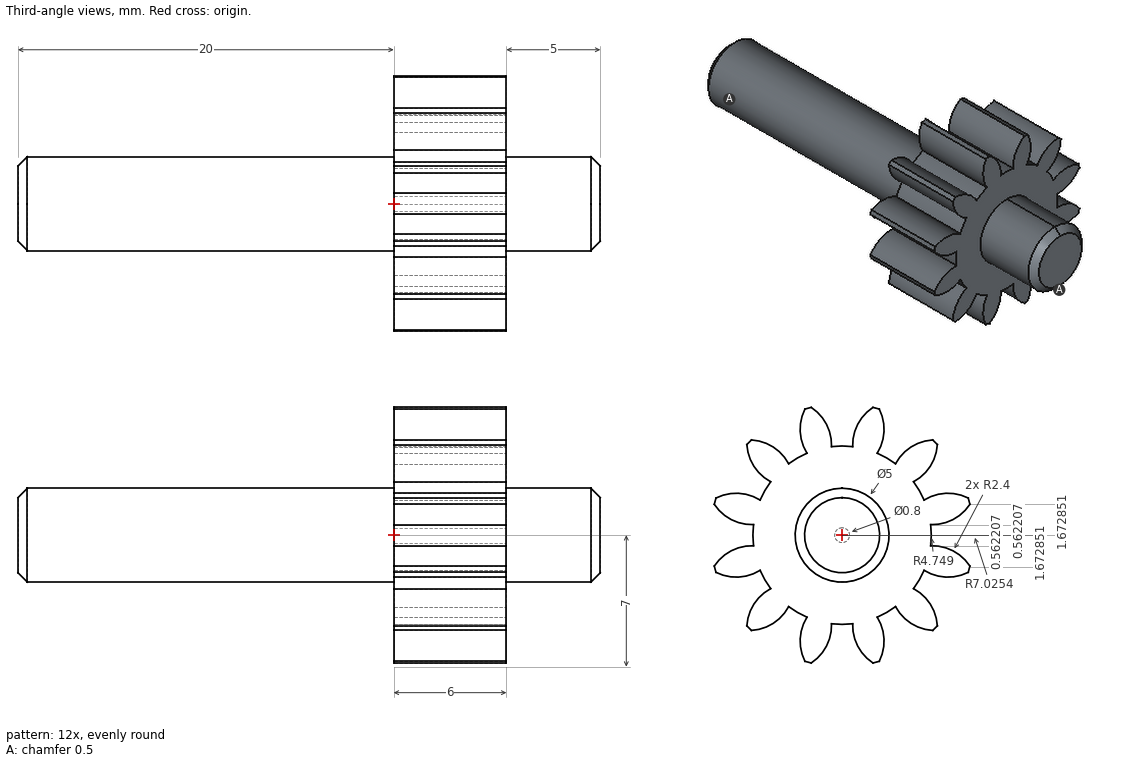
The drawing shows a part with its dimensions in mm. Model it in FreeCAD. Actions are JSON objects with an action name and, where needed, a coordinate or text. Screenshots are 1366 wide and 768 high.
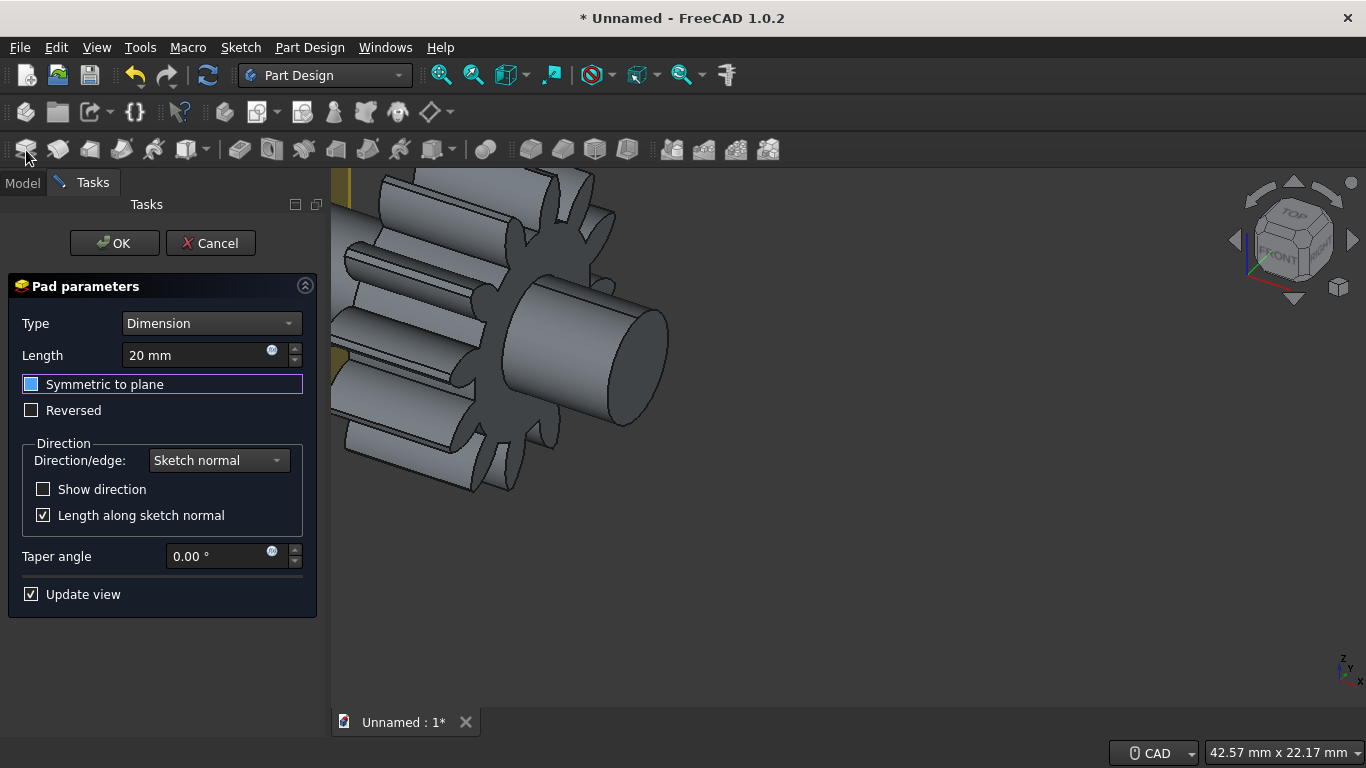
{"action": "left_click", "coordinate": [115, 243]}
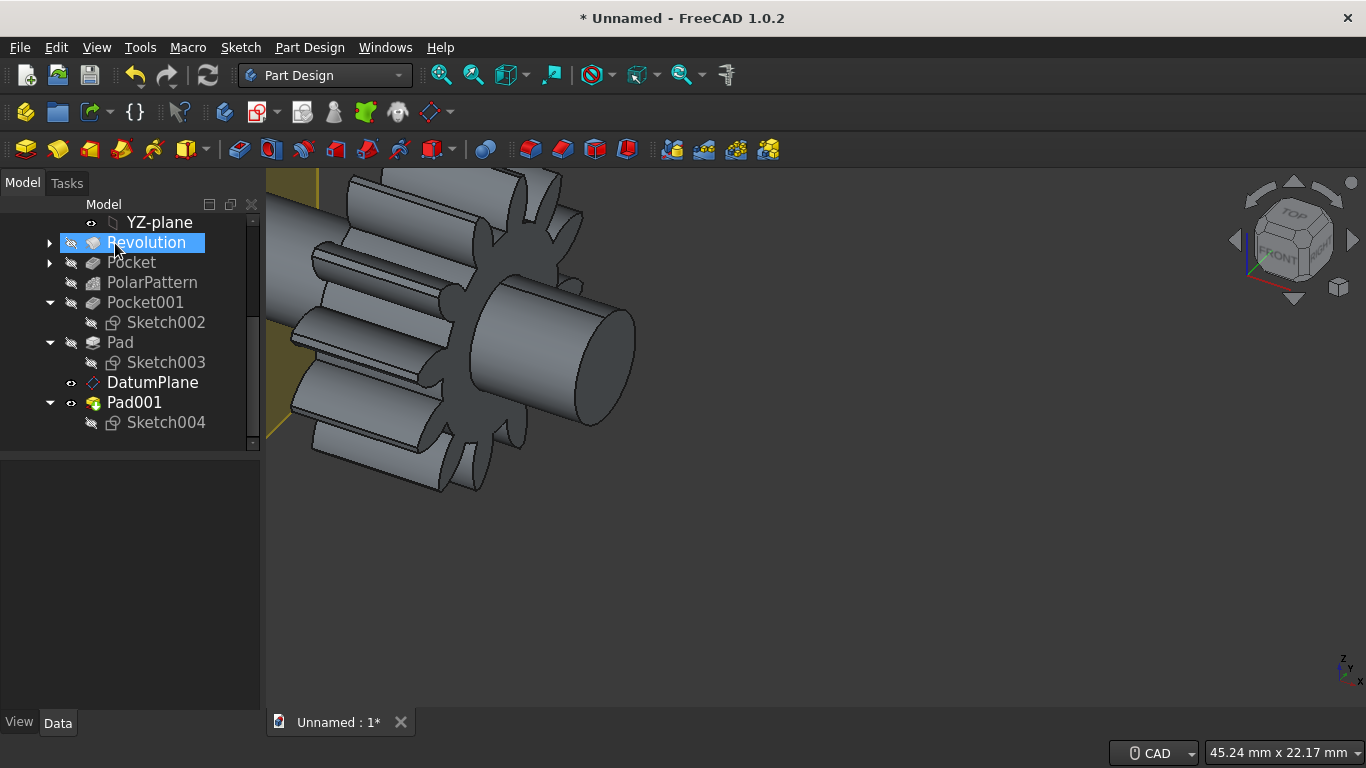
{"action": "left_click", "coordinate": [116, 383]}
{"action": "key", "text": "space"}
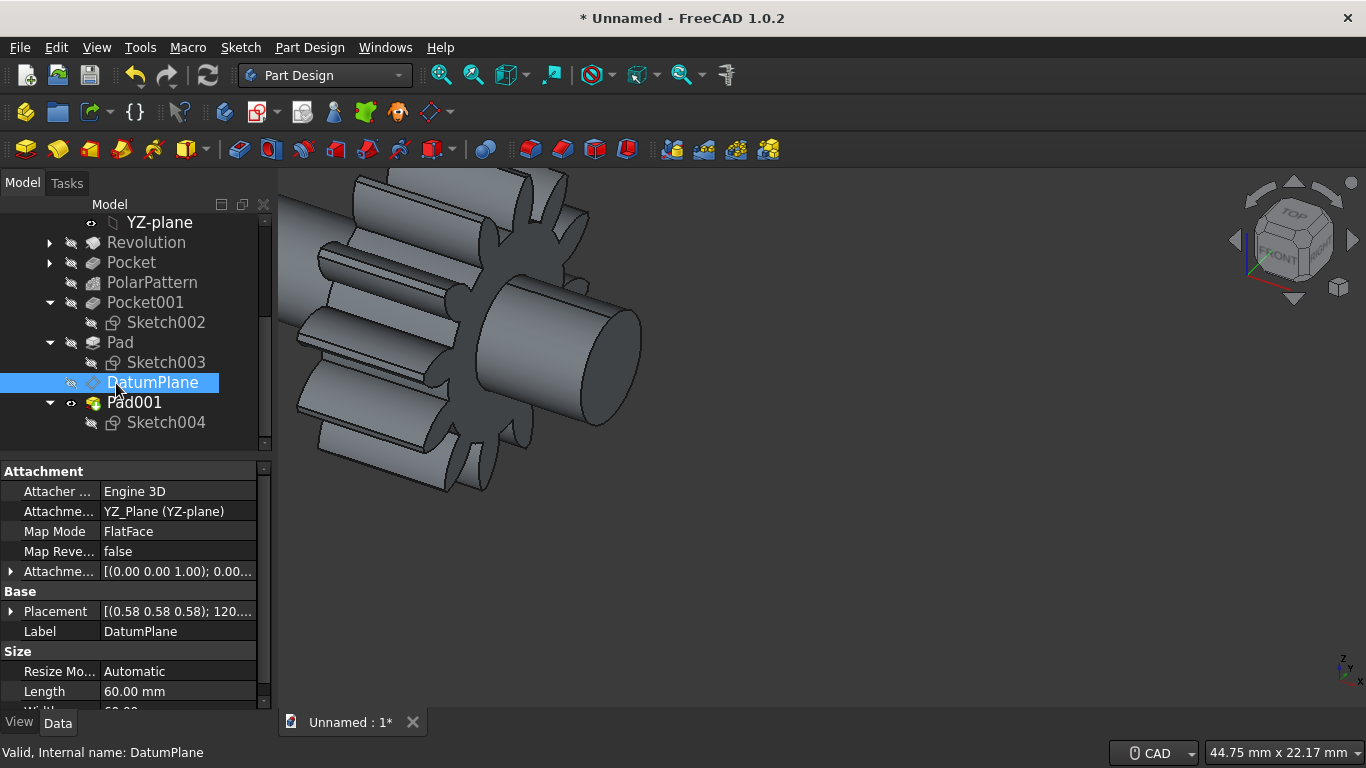
{"action": "left_click", "coordinate": [442, 76]}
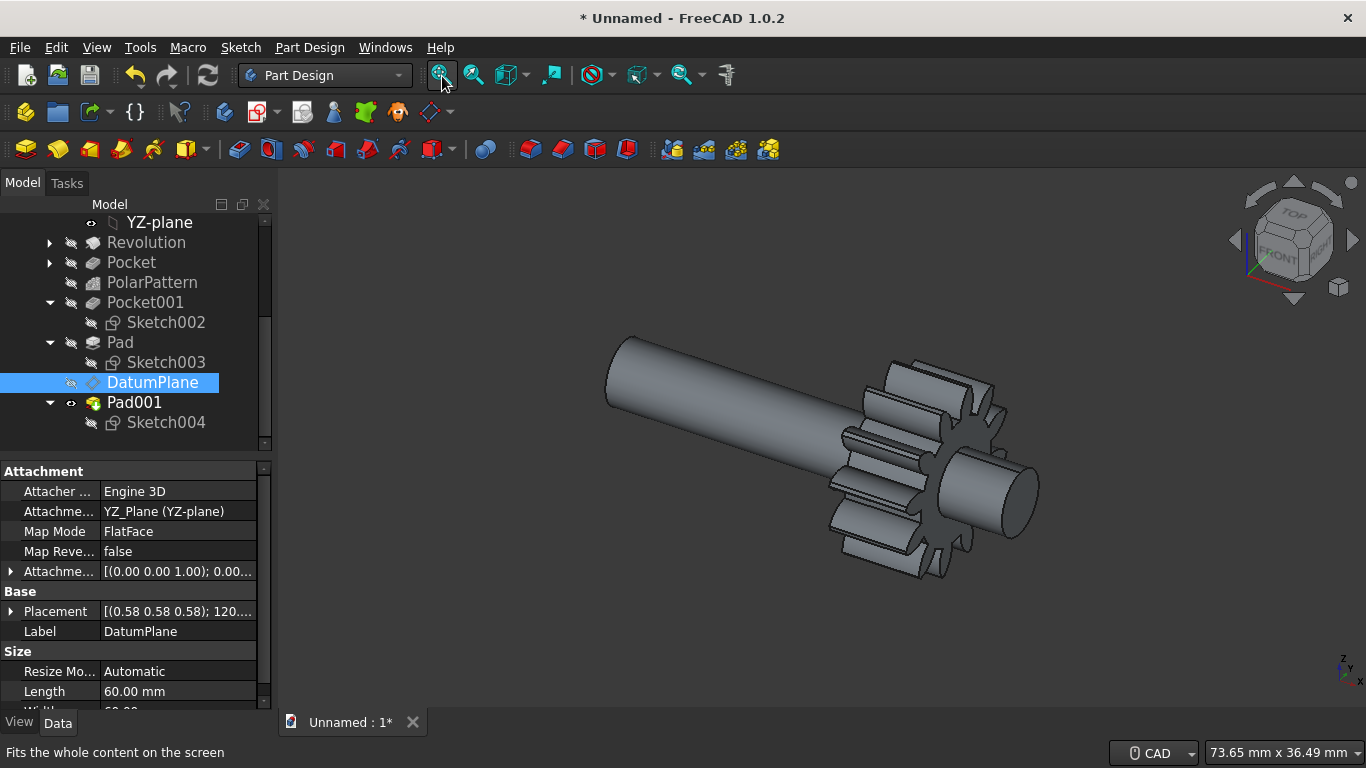
{"action": "left_click", "coordinate": [1009, 537]}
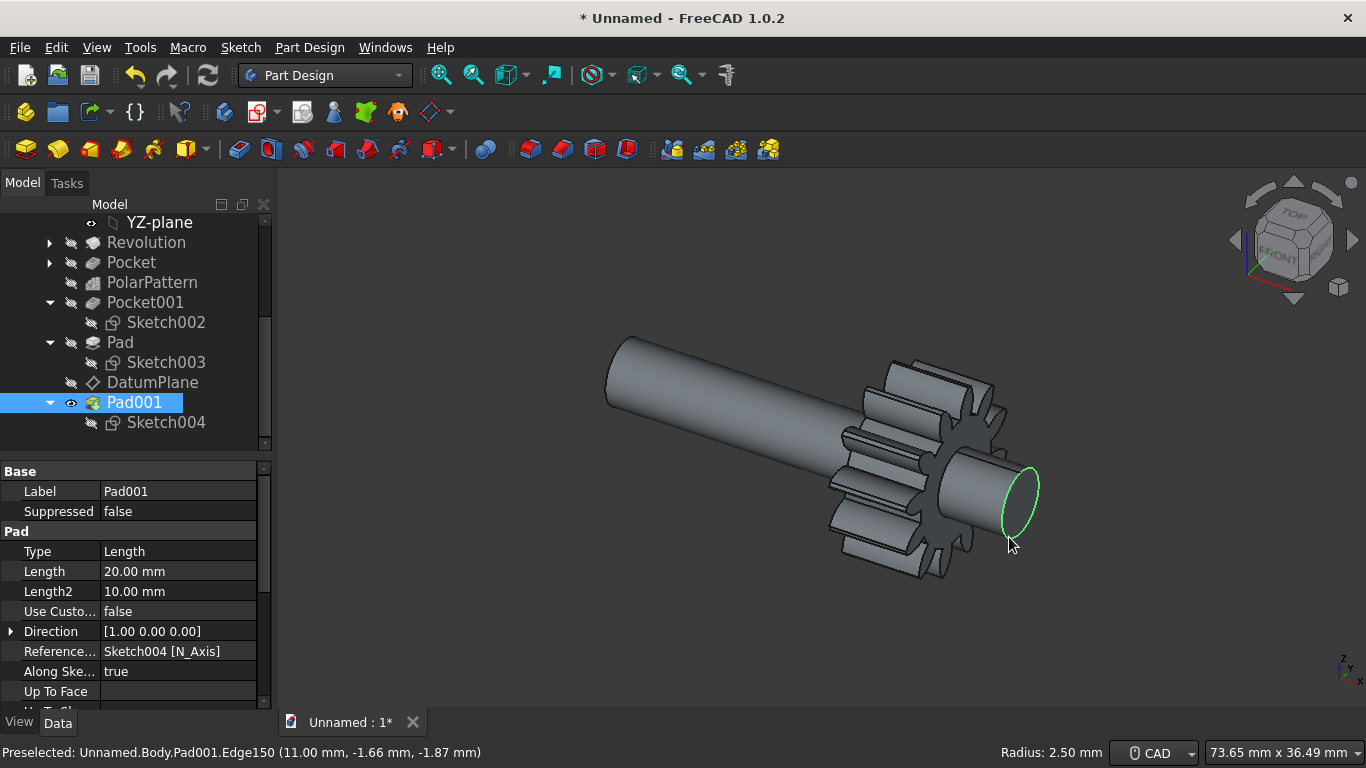
{"action": "key", "text": "0"}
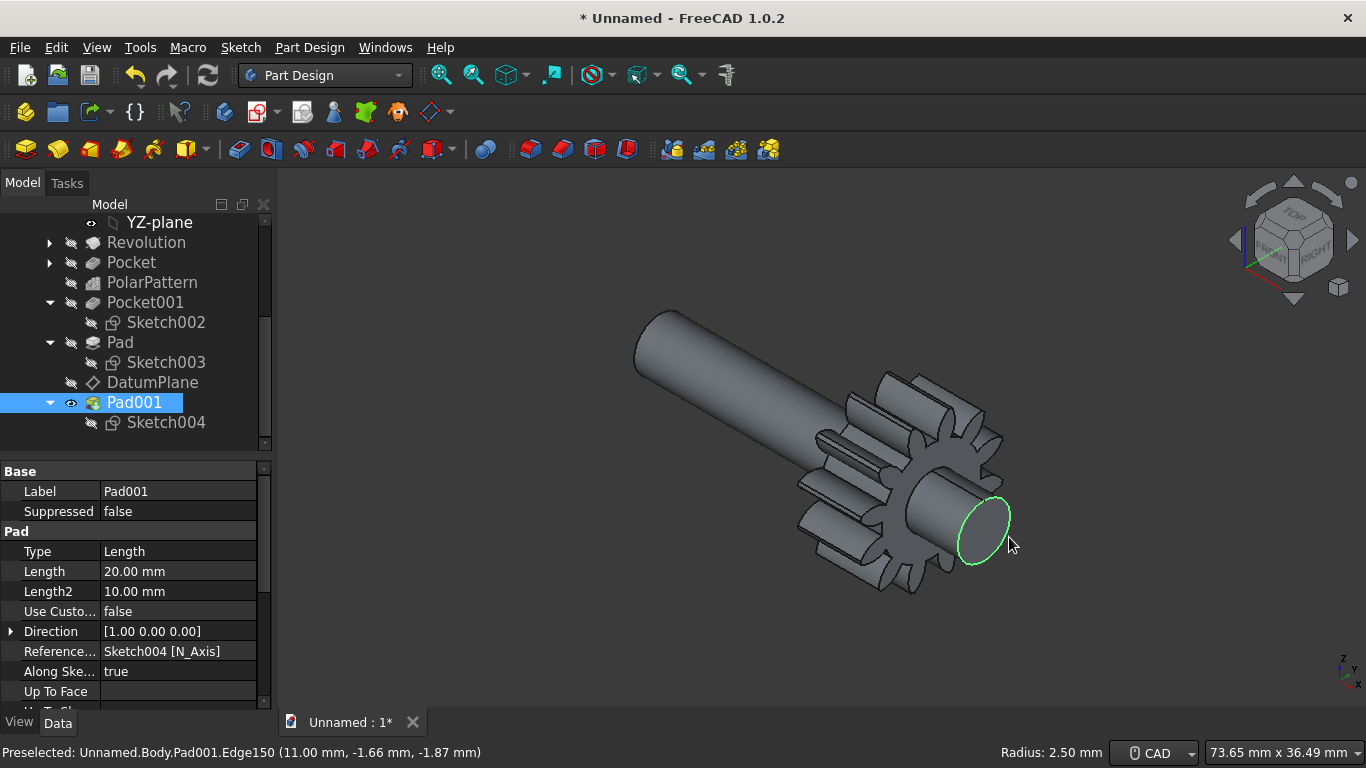
{"action": "key", "text": "2"}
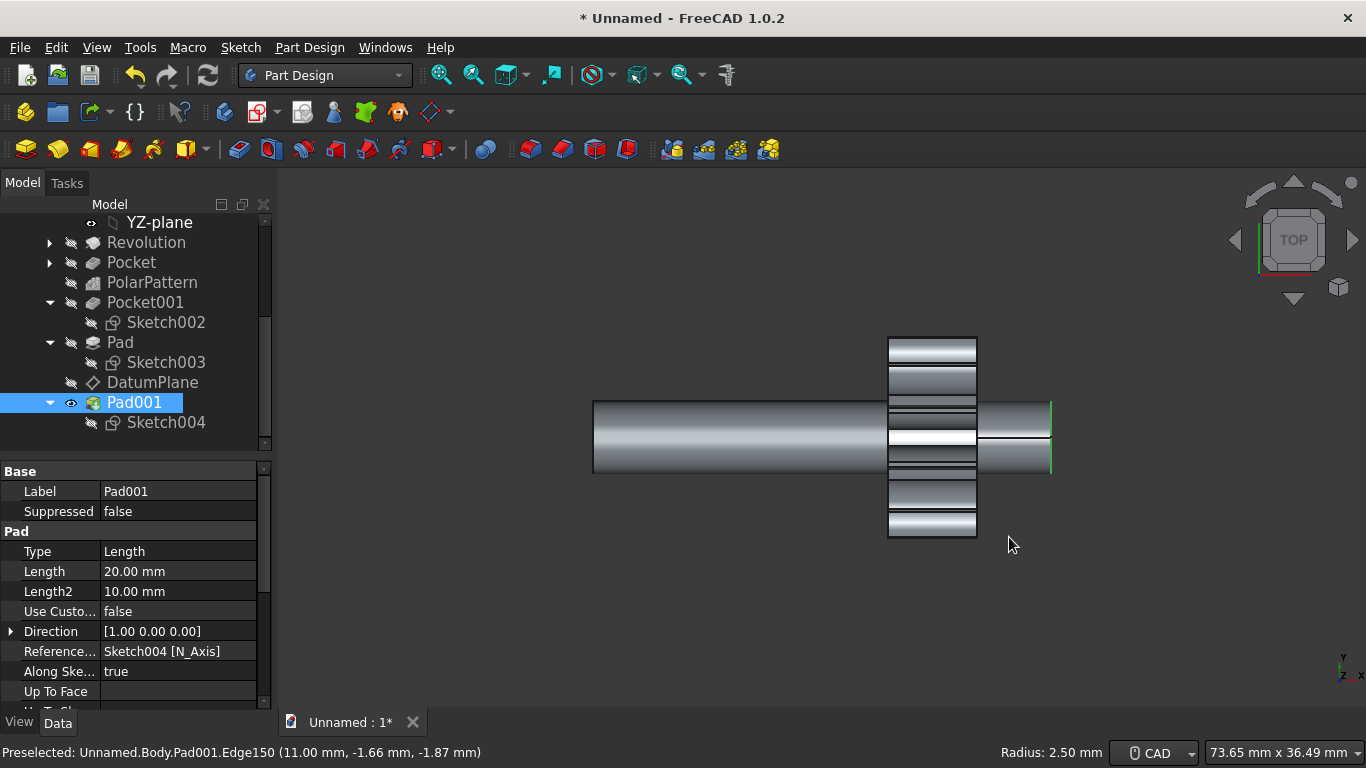
{"action": "left_click", "coordinate": [442, 76]}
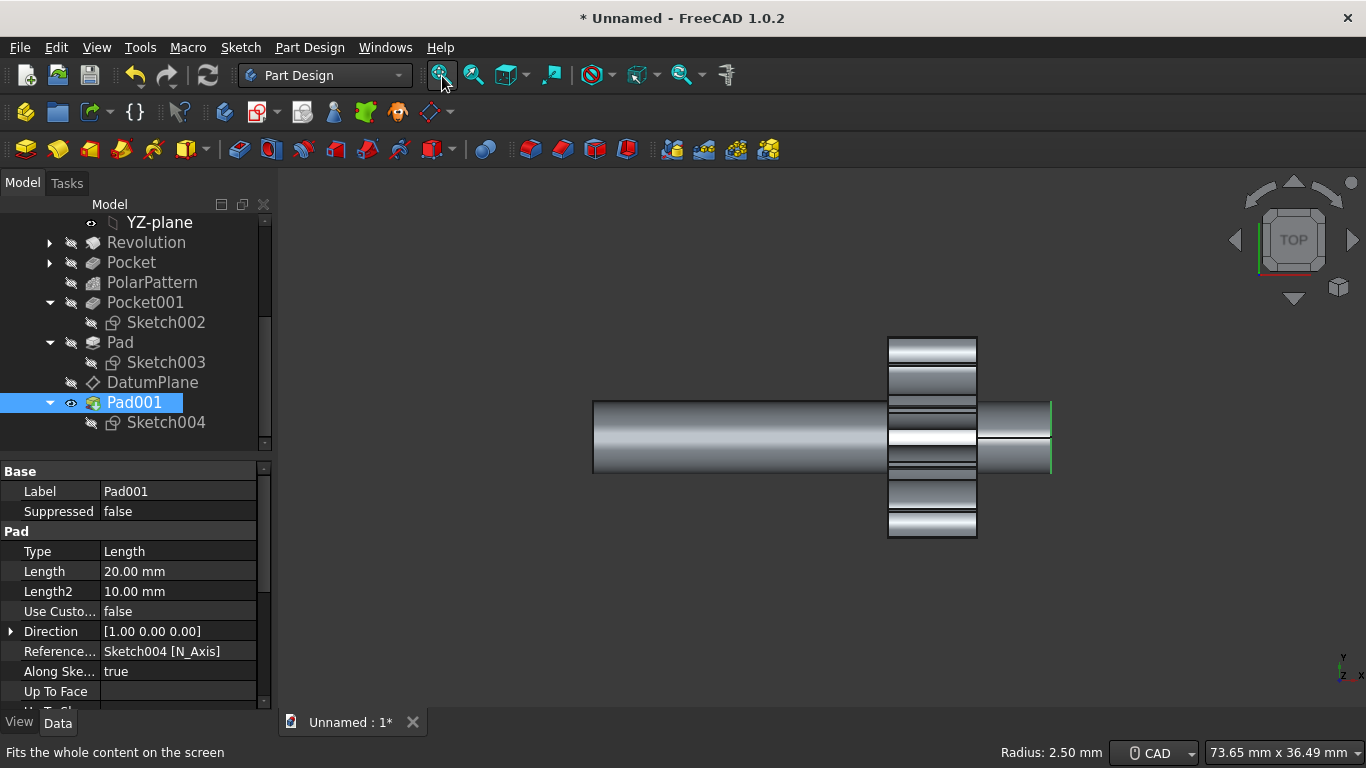
{"action": "left_click", "coordinate": [593, 473], "text": "ctrl"}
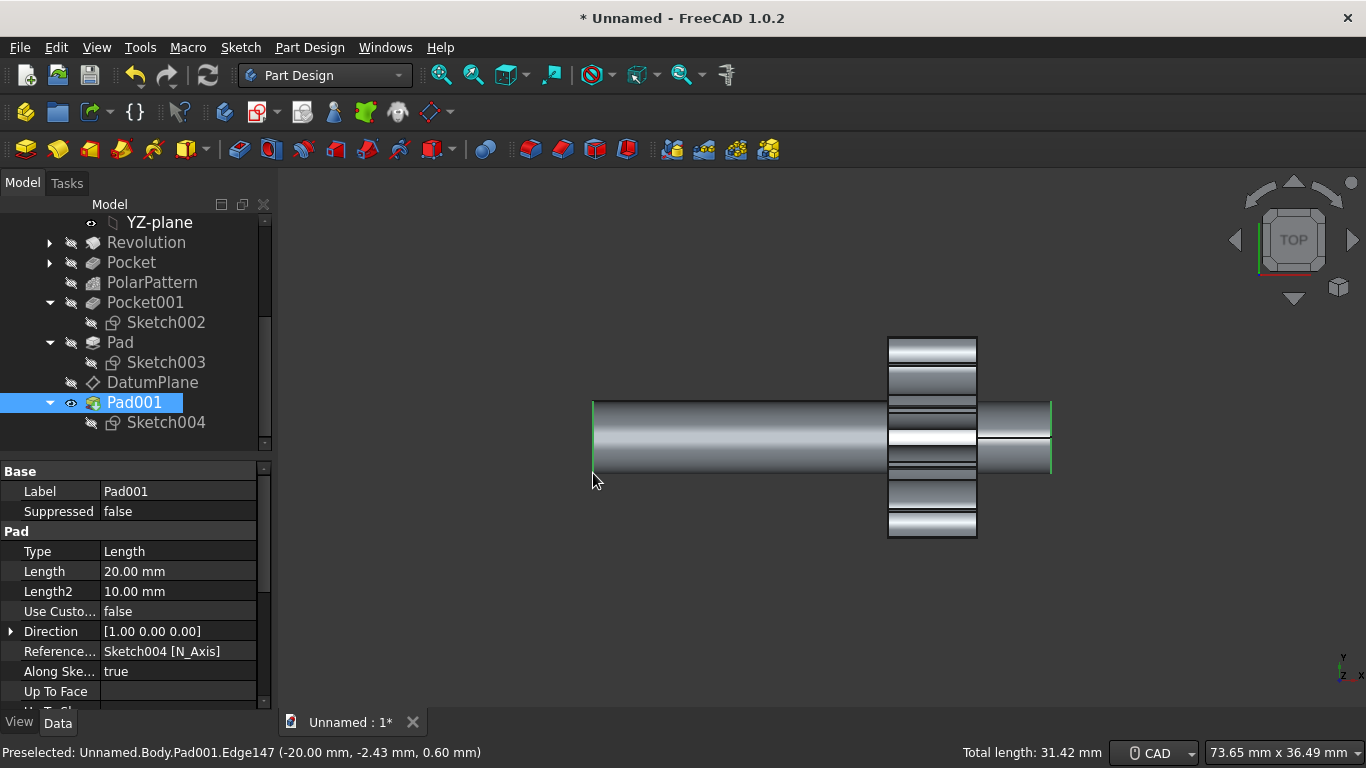
{"action": "left_click", "coordinate": [564, 150]}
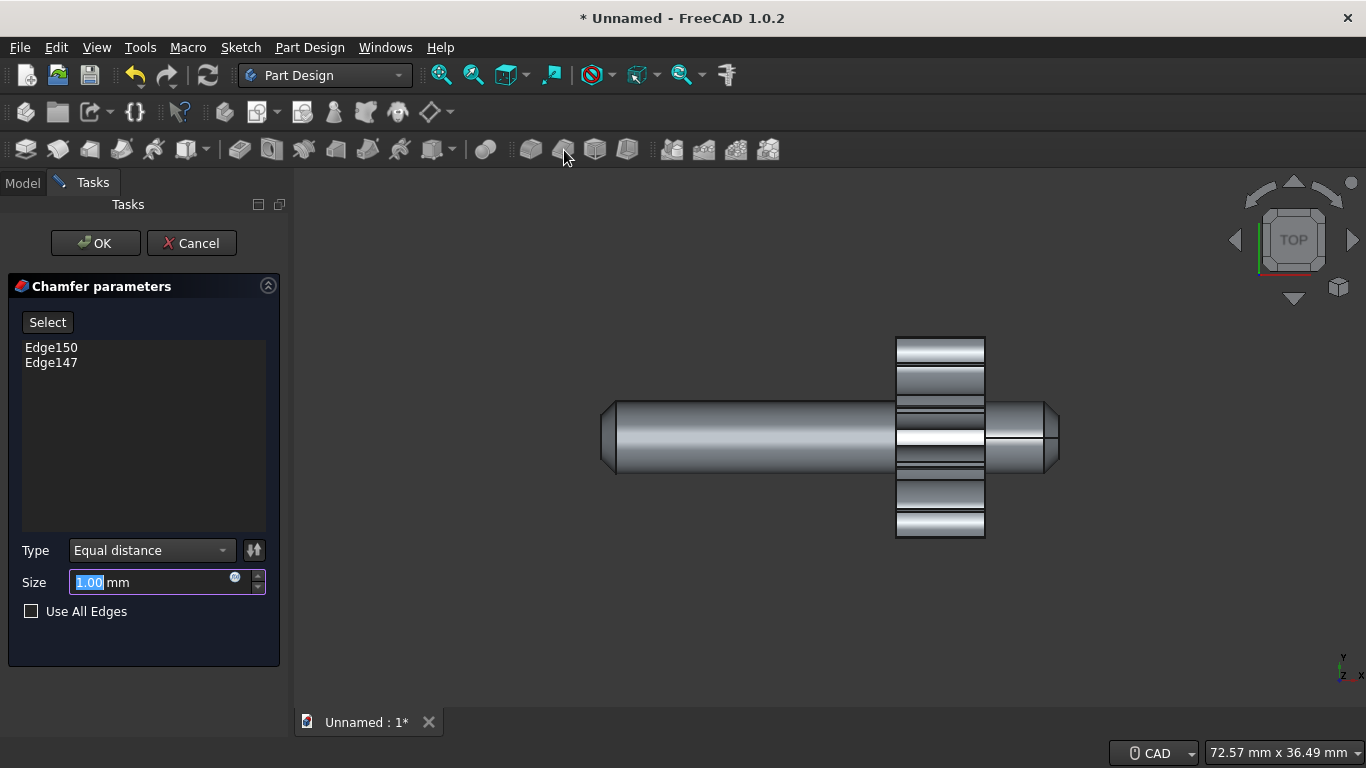
{"action": "type", "text": "0.5"}
{"action": "key", "text": "Tab"}